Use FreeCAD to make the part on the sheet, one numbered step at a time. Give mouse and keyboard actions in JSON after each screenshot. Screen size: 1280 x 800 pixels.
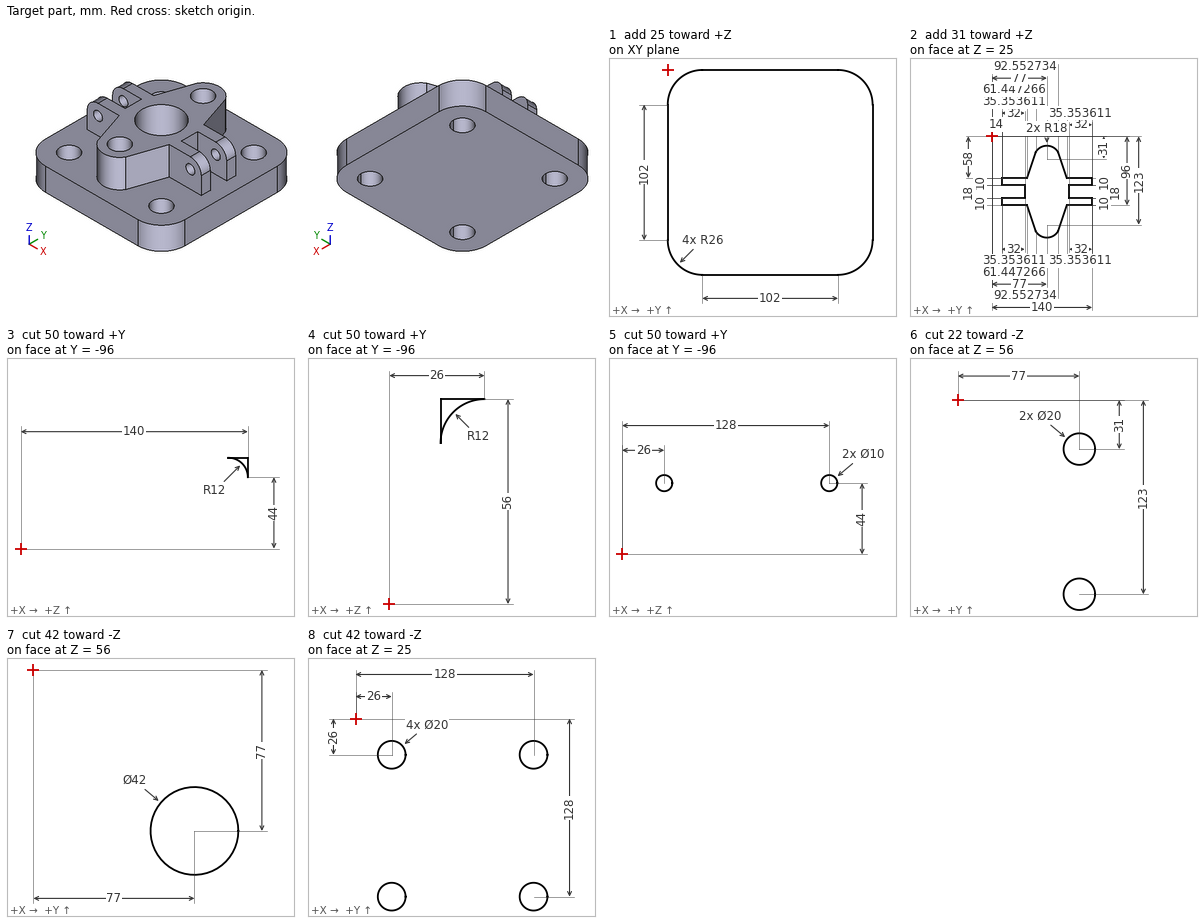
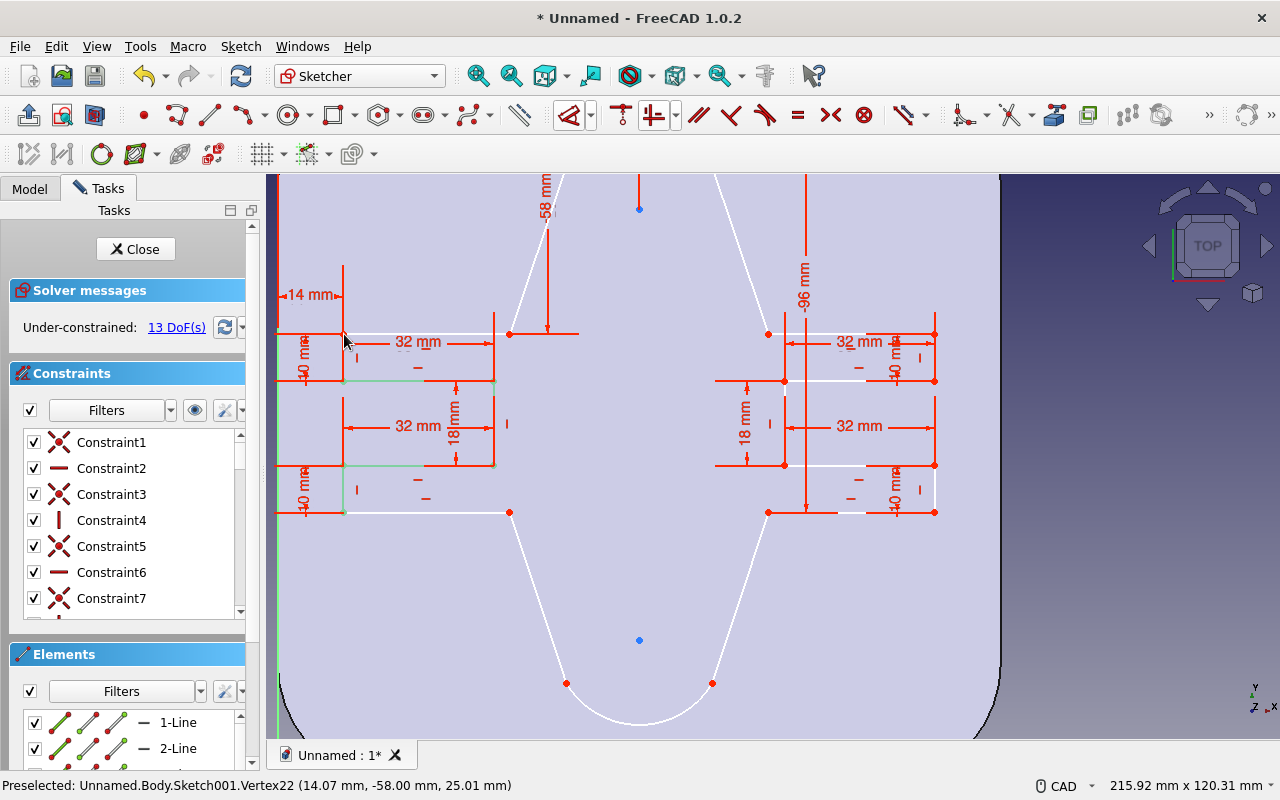
{"action": "left_click", "coordinate": [639, 210]}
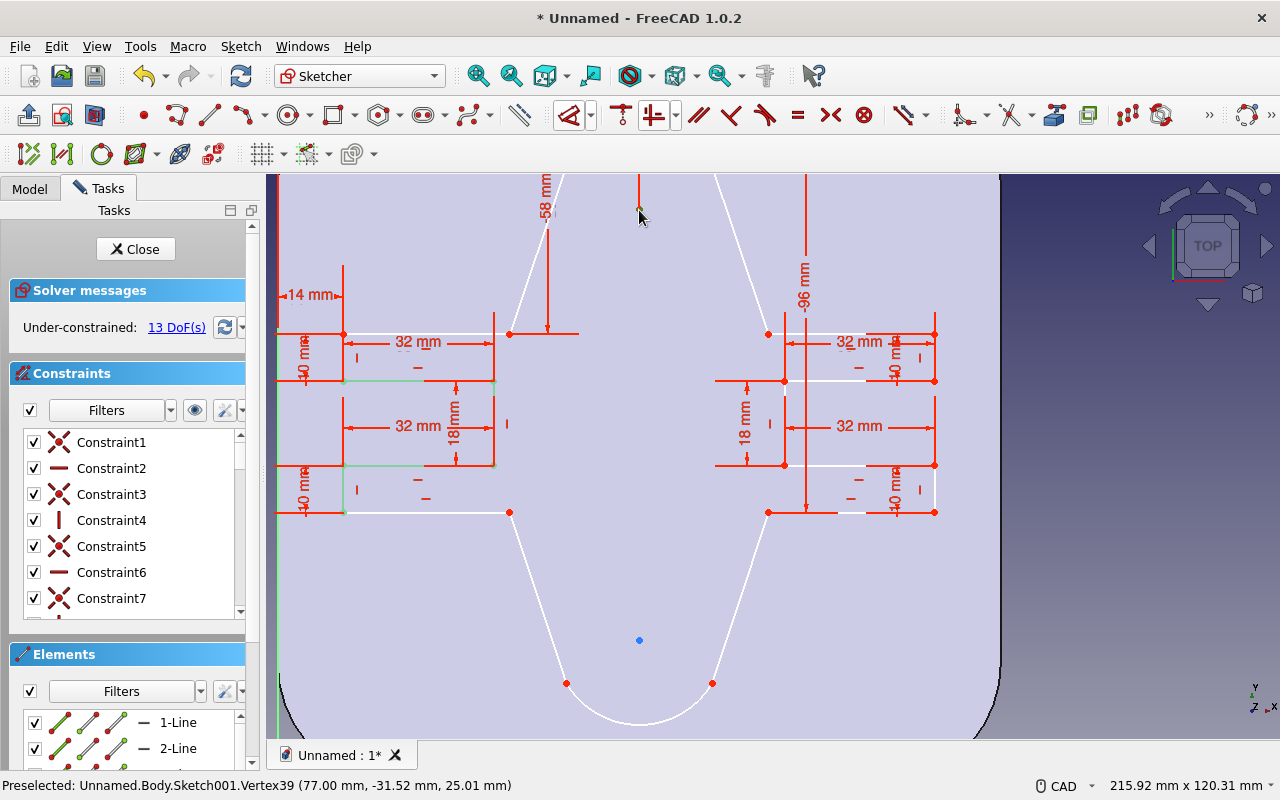
{"action": "key", "text": "l"}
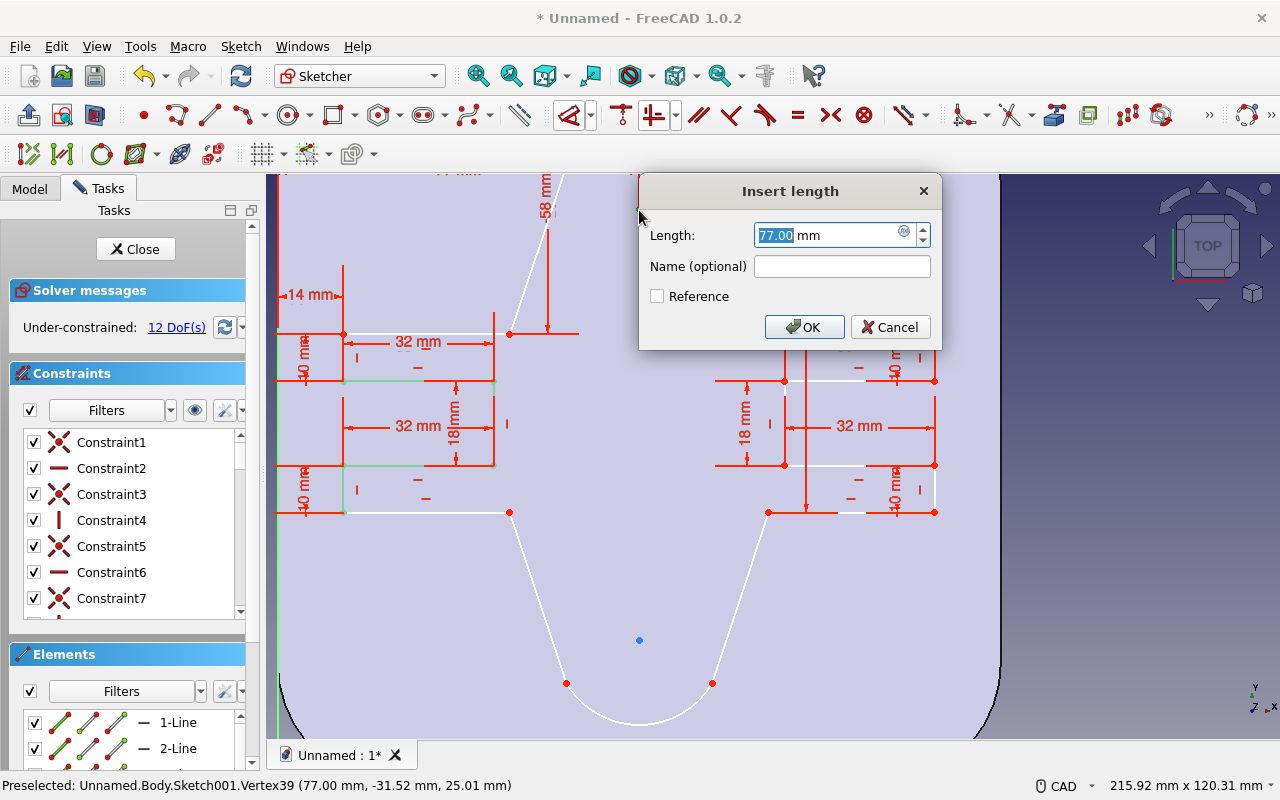
{"action": "type", "text": "77"}
{"action": "key", "text": "Return"}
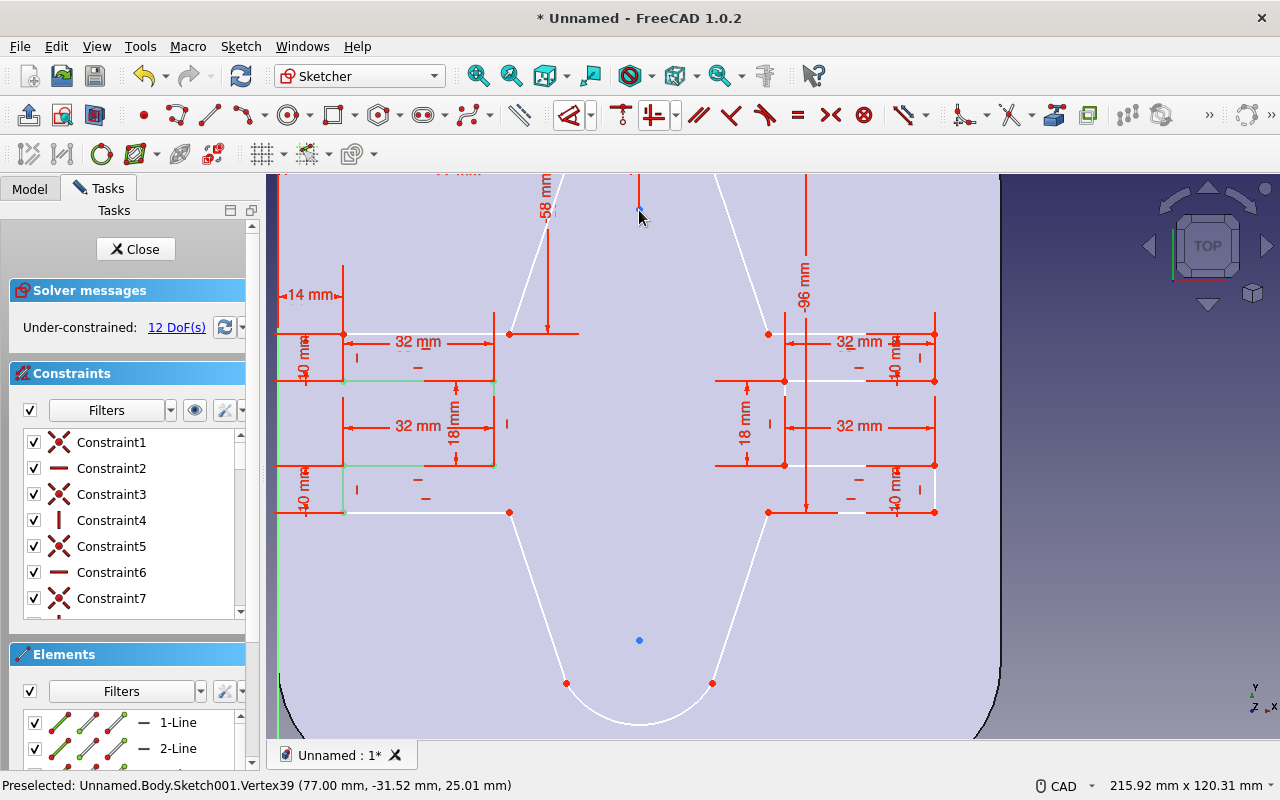
{"action": "left_click", "coordinate": [639, 210]}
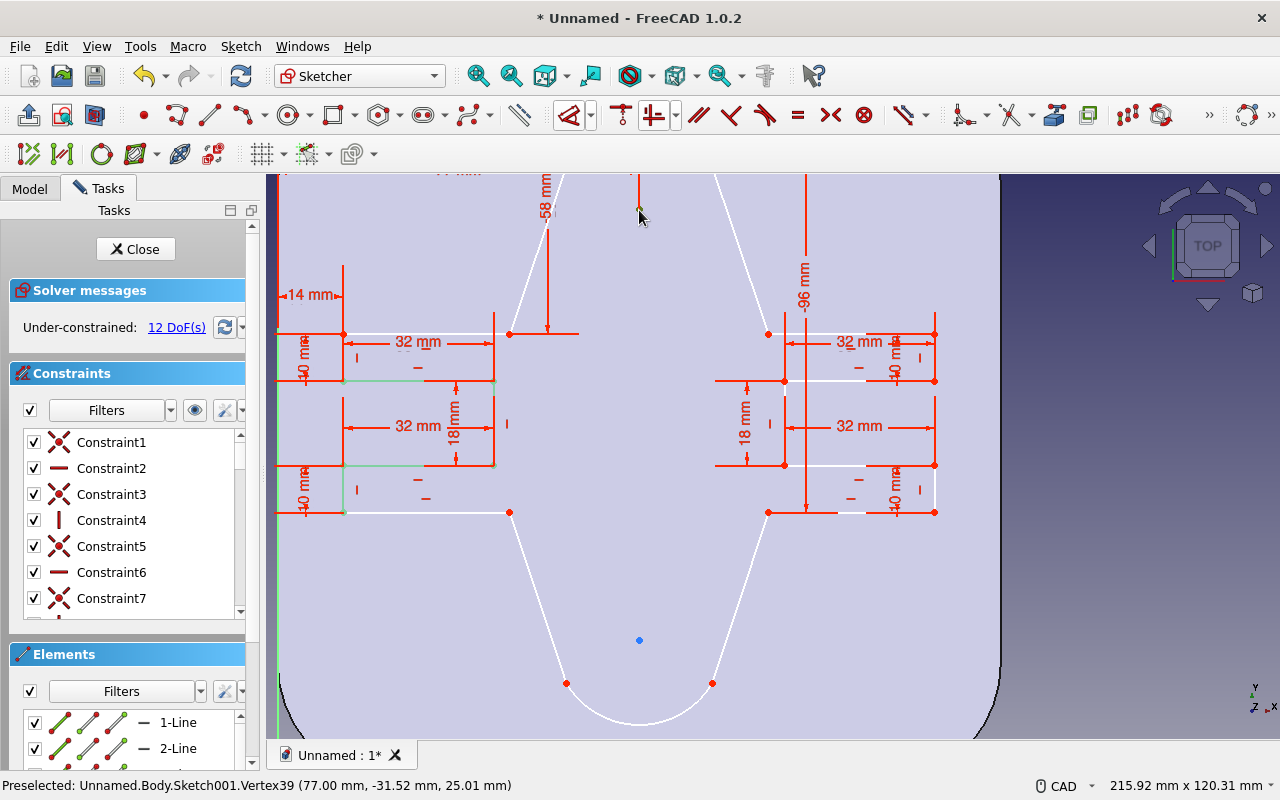
{"action": "key", "text": "i"}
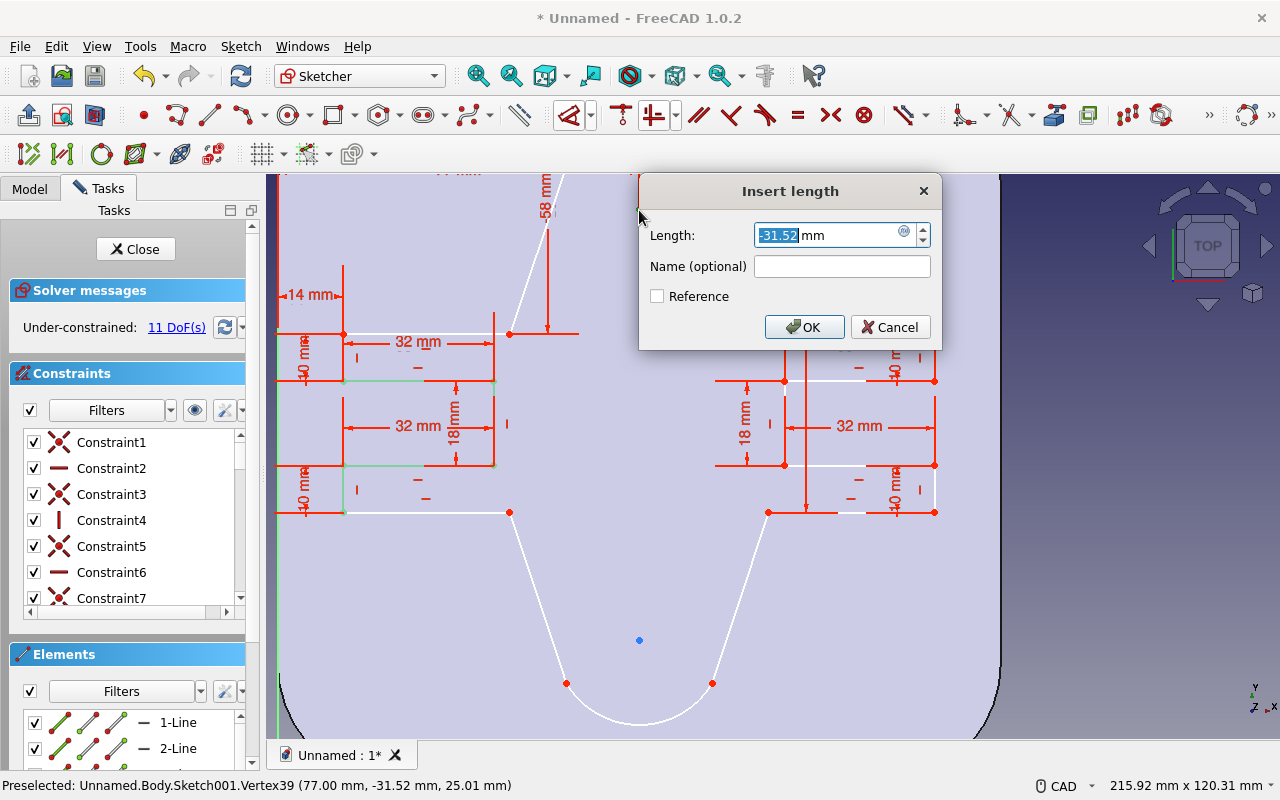
{"action": "type", "text": "-31"}
{"action": "key", "text": "Return"}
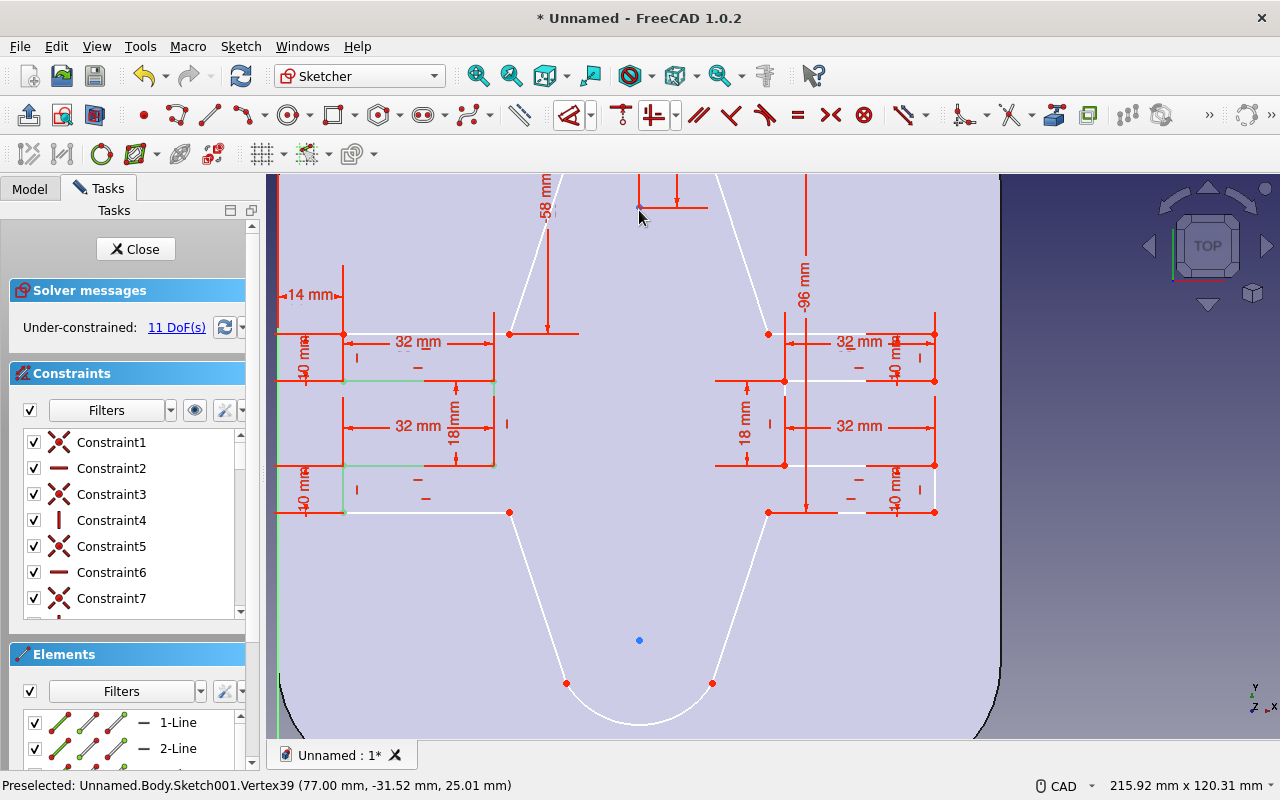
{"action": "left_click", "coordinate": [639, 640]}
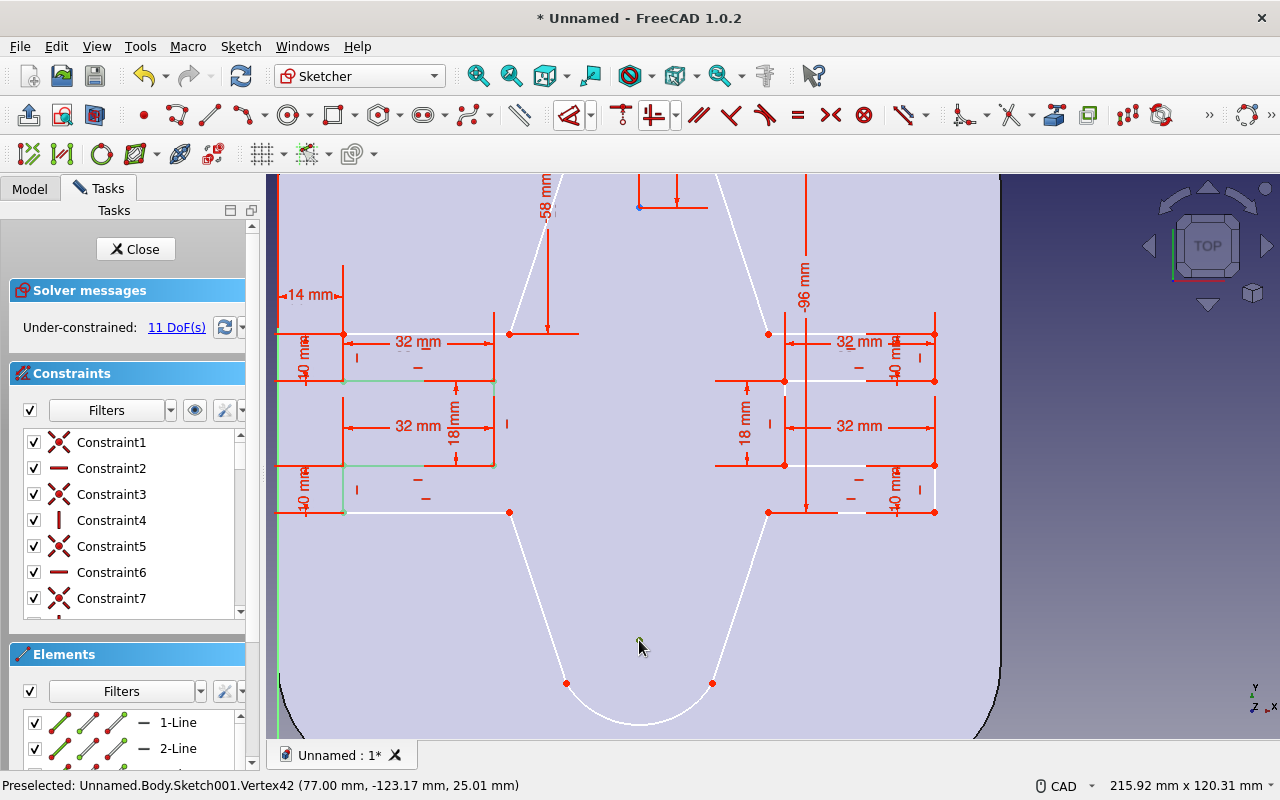
{"action": "left_click", "coordinate": [590, 116]}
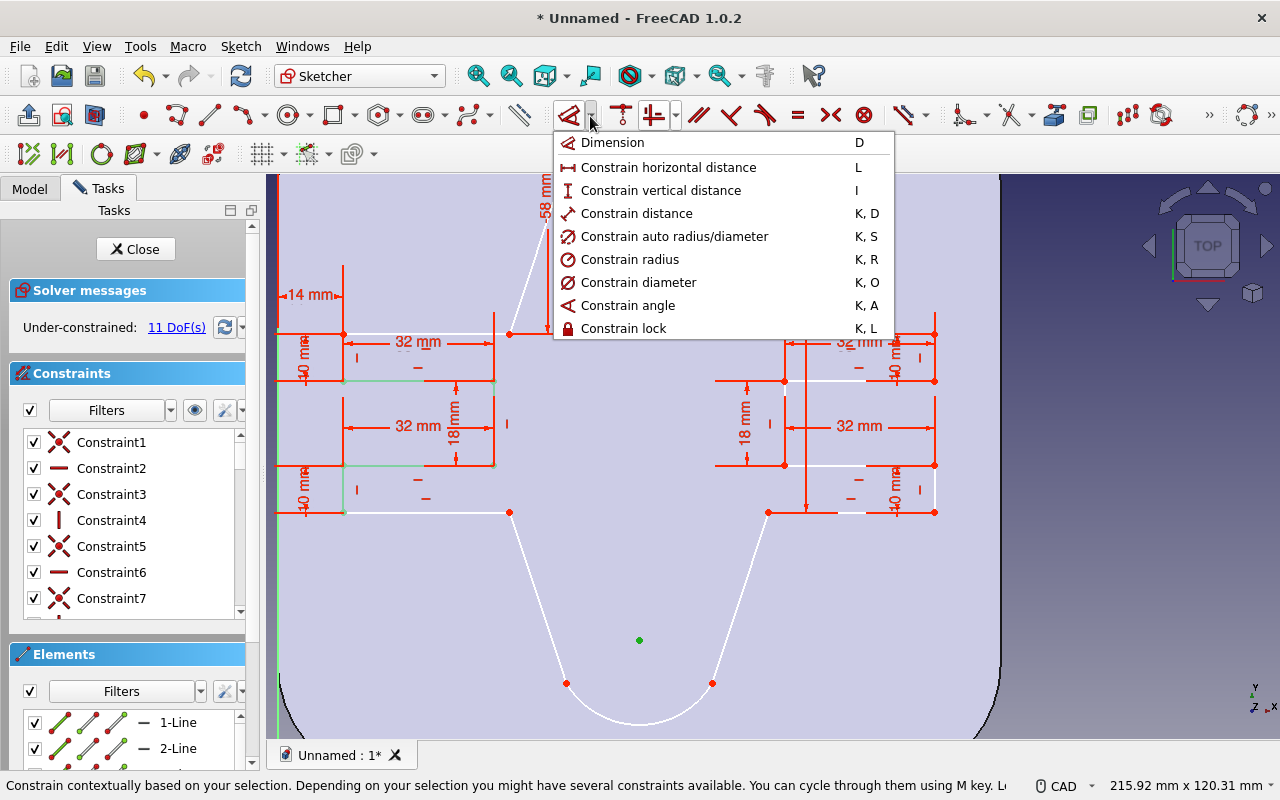
{"action": "left_click", "coordinate": [724, 168]}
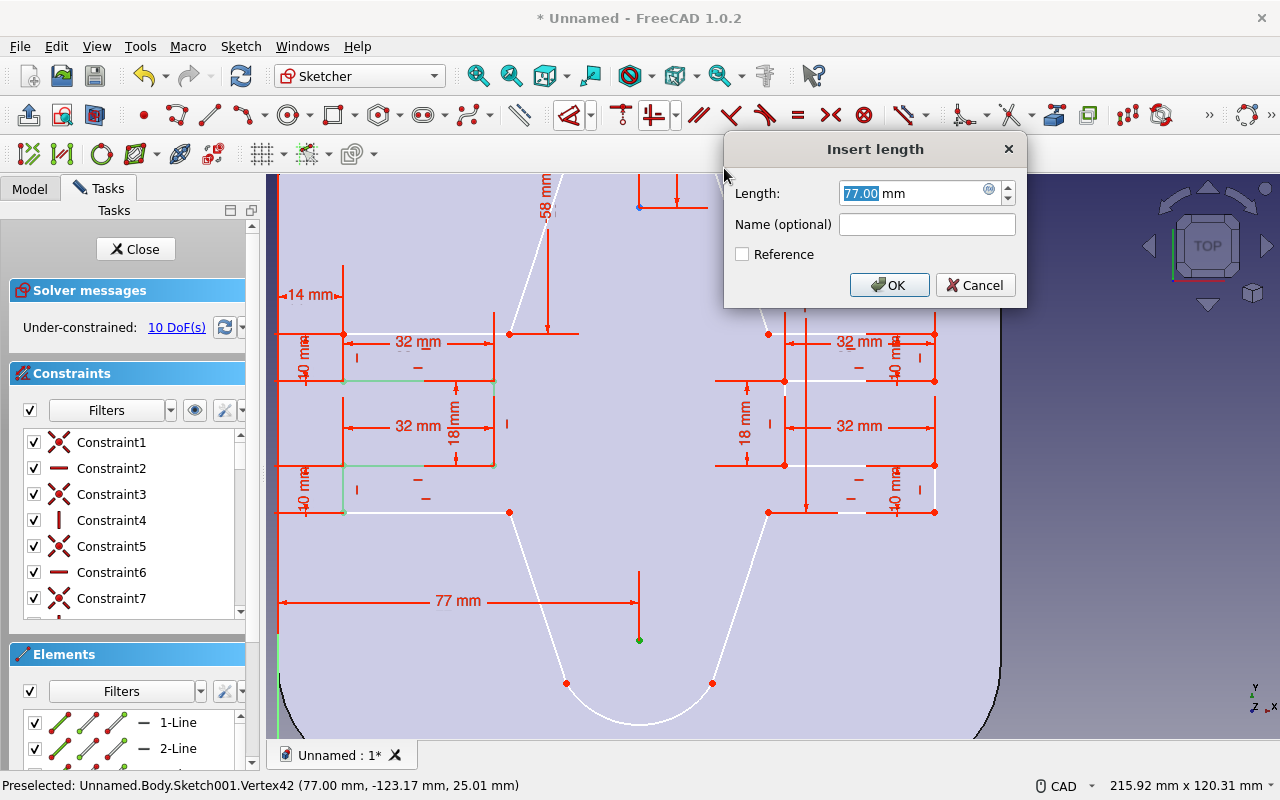
{"action": "type", "text": "77"}
{"action": "key", "text": "Return"}